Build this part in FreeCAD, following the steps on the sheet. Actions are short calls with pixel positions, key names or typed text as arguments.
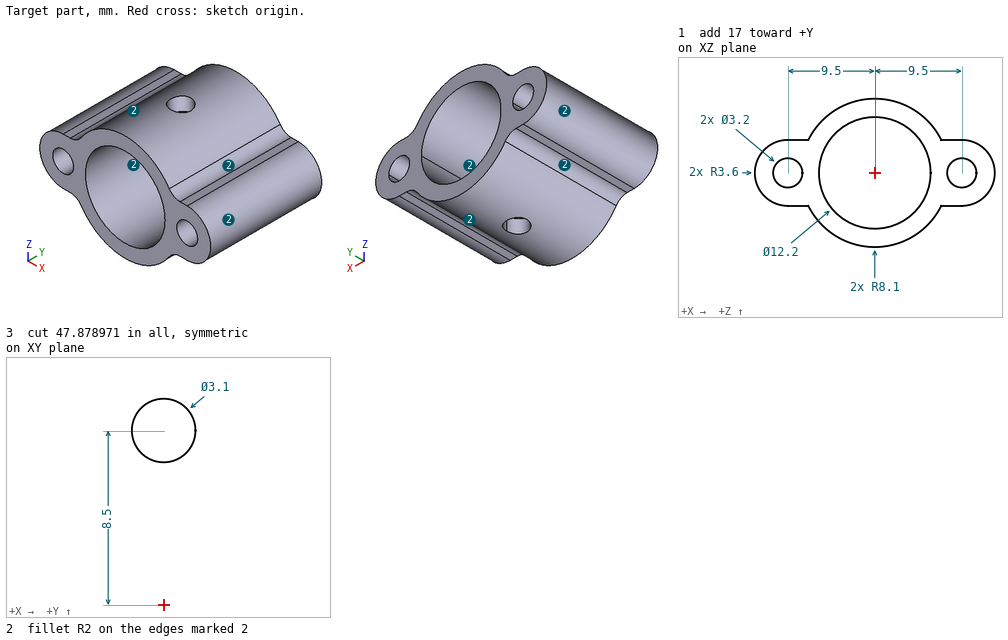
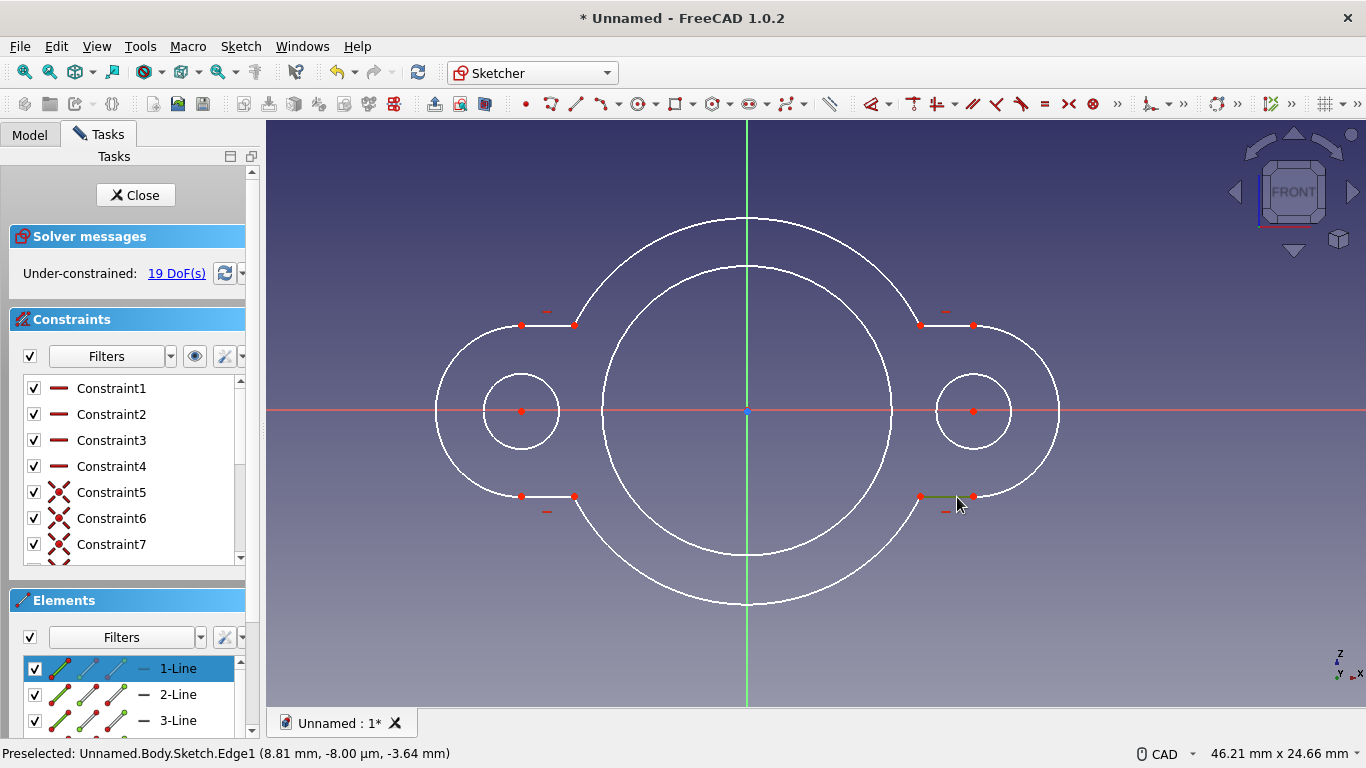
click(1043, 462)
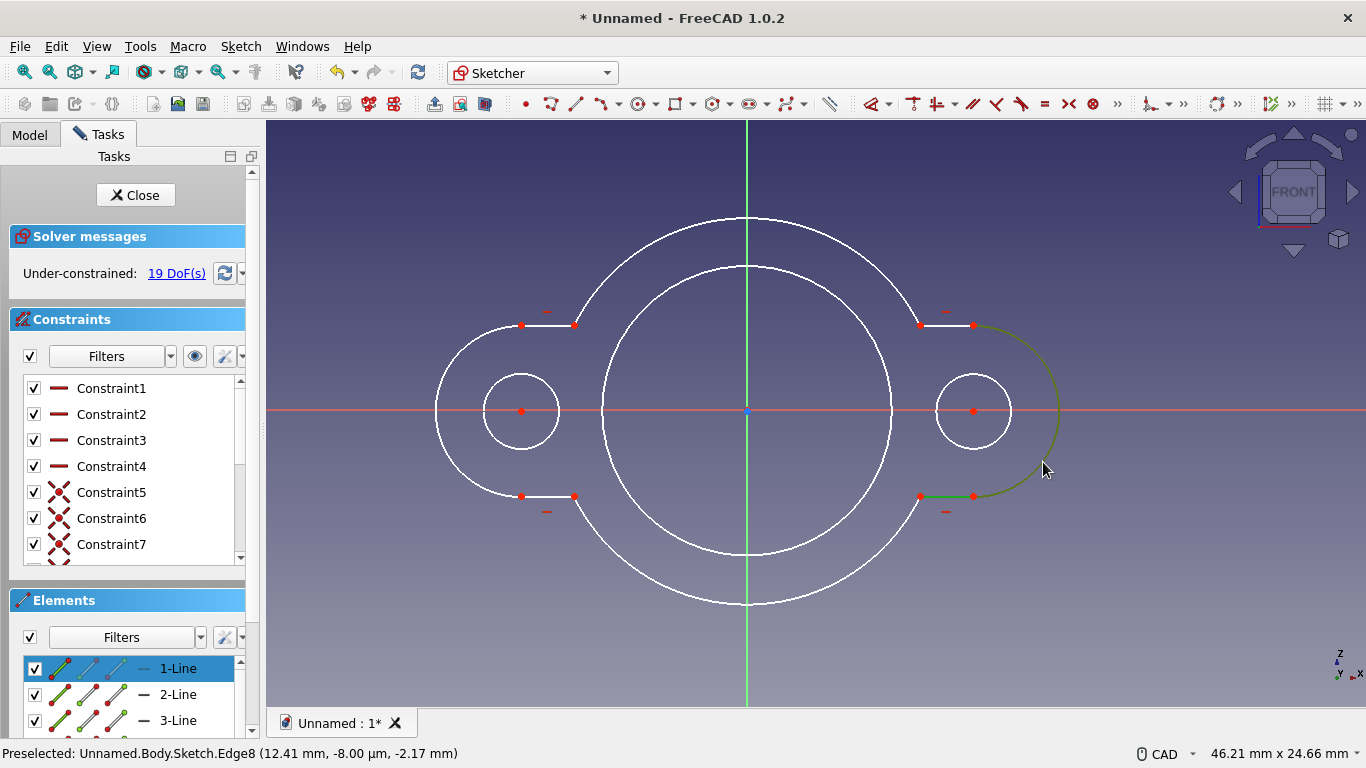
key(t)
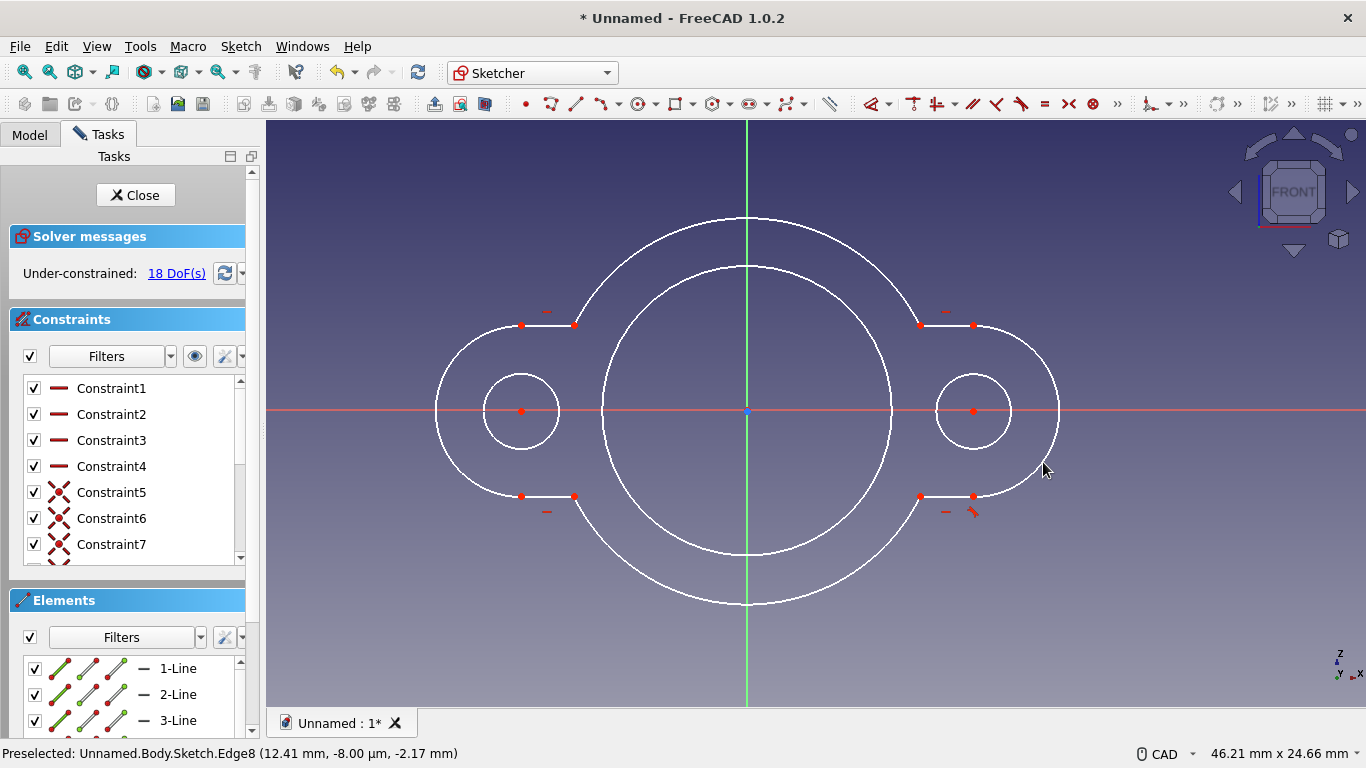
click(558, 497)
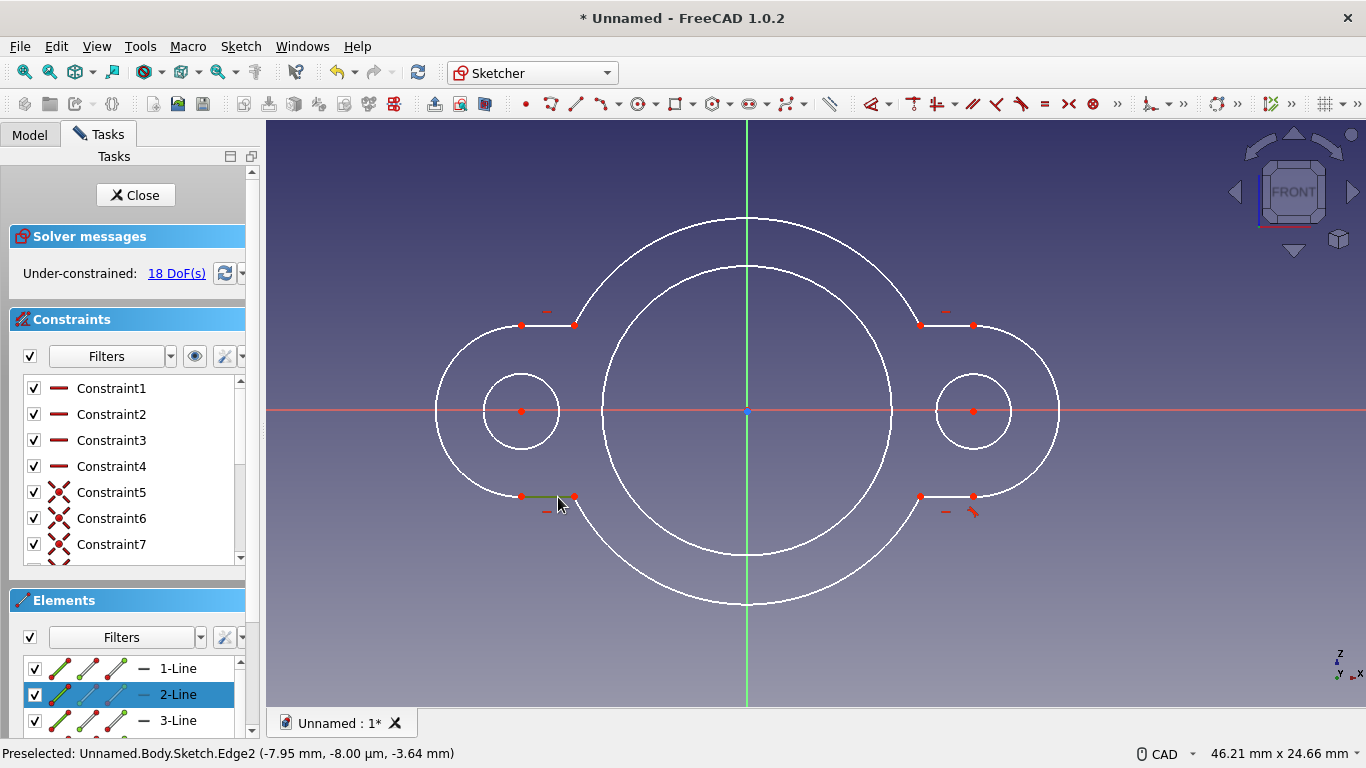
click(452, 361)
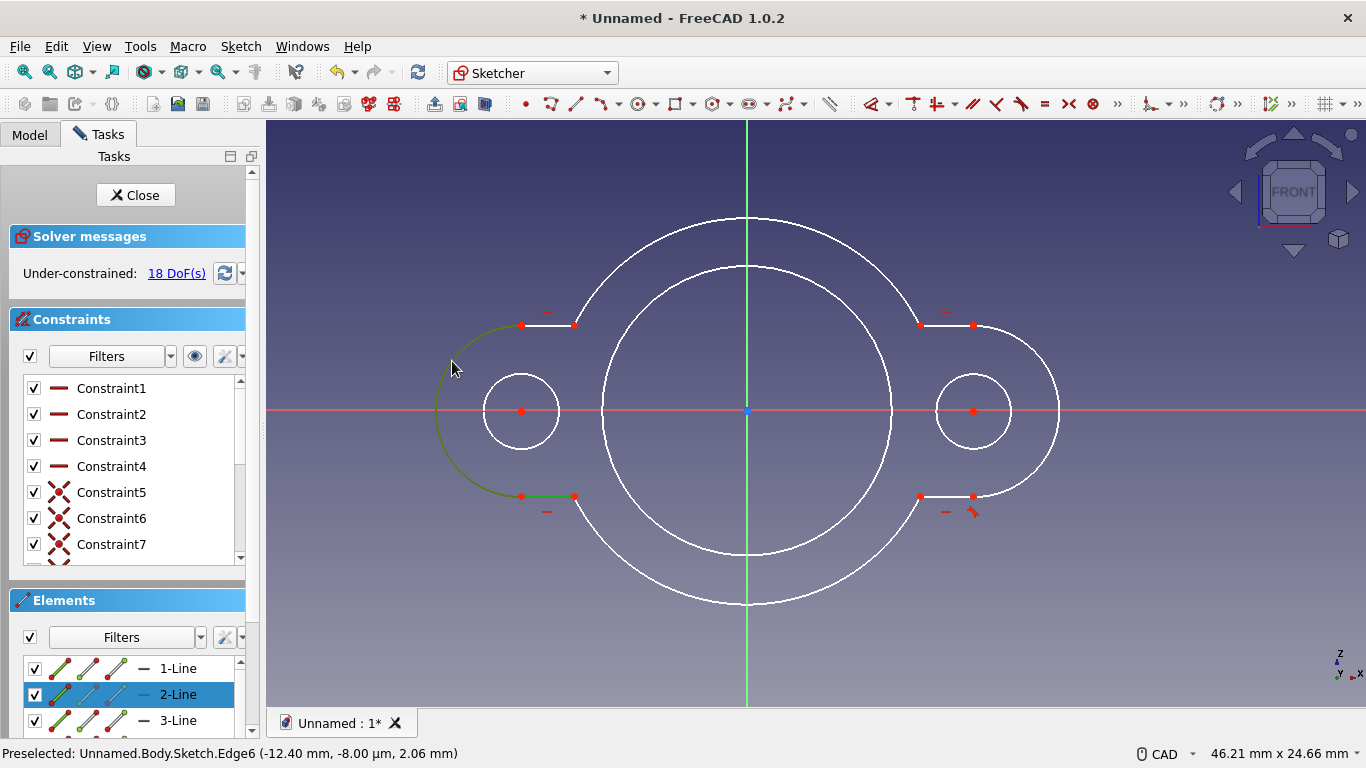
key(t)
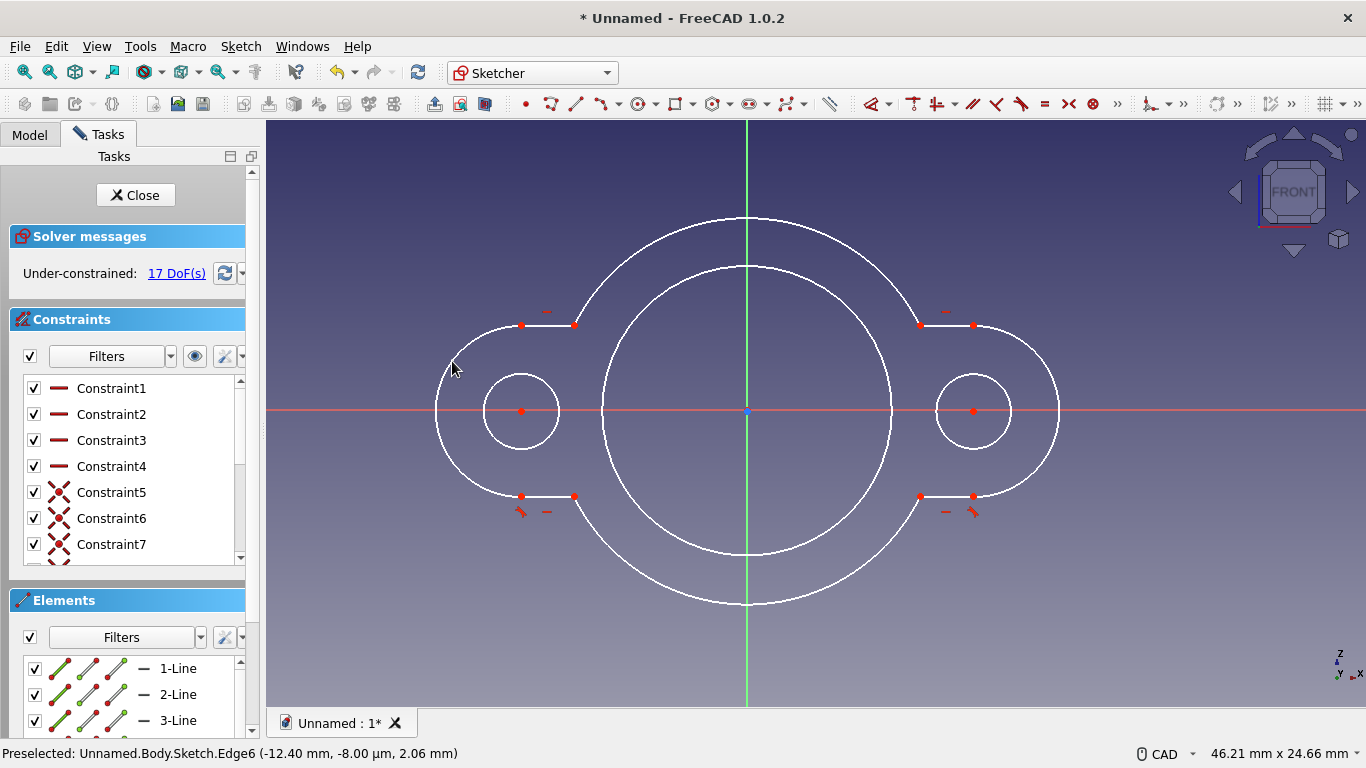
click(537, 326)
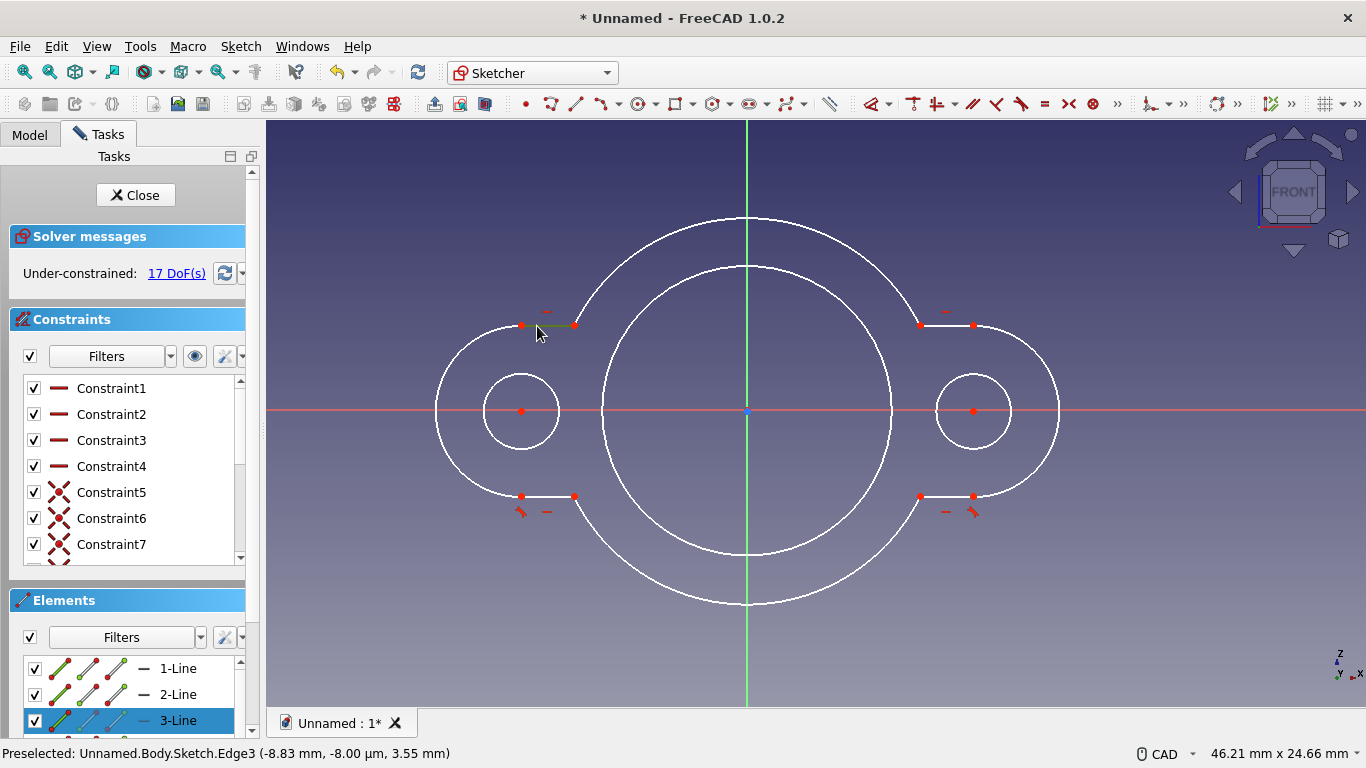
click(452, 361)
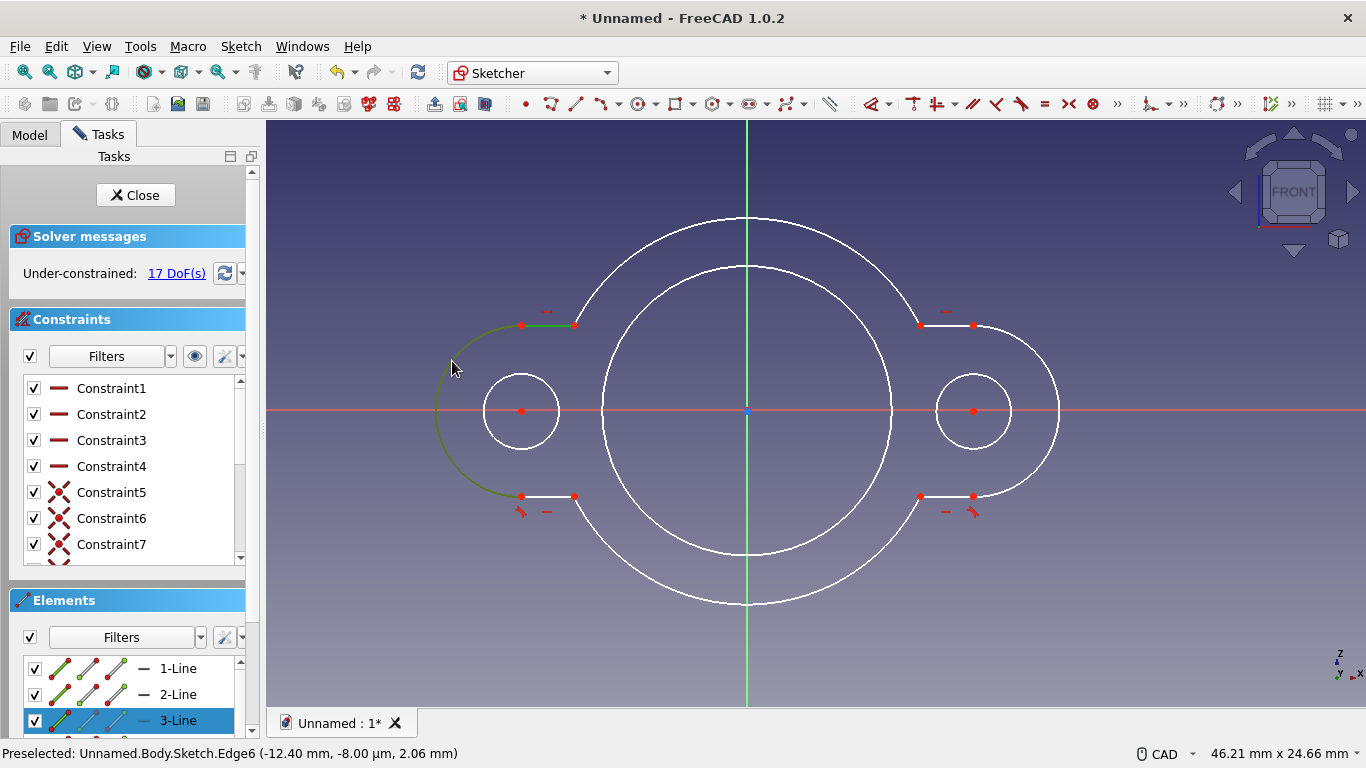
click(1021, 104)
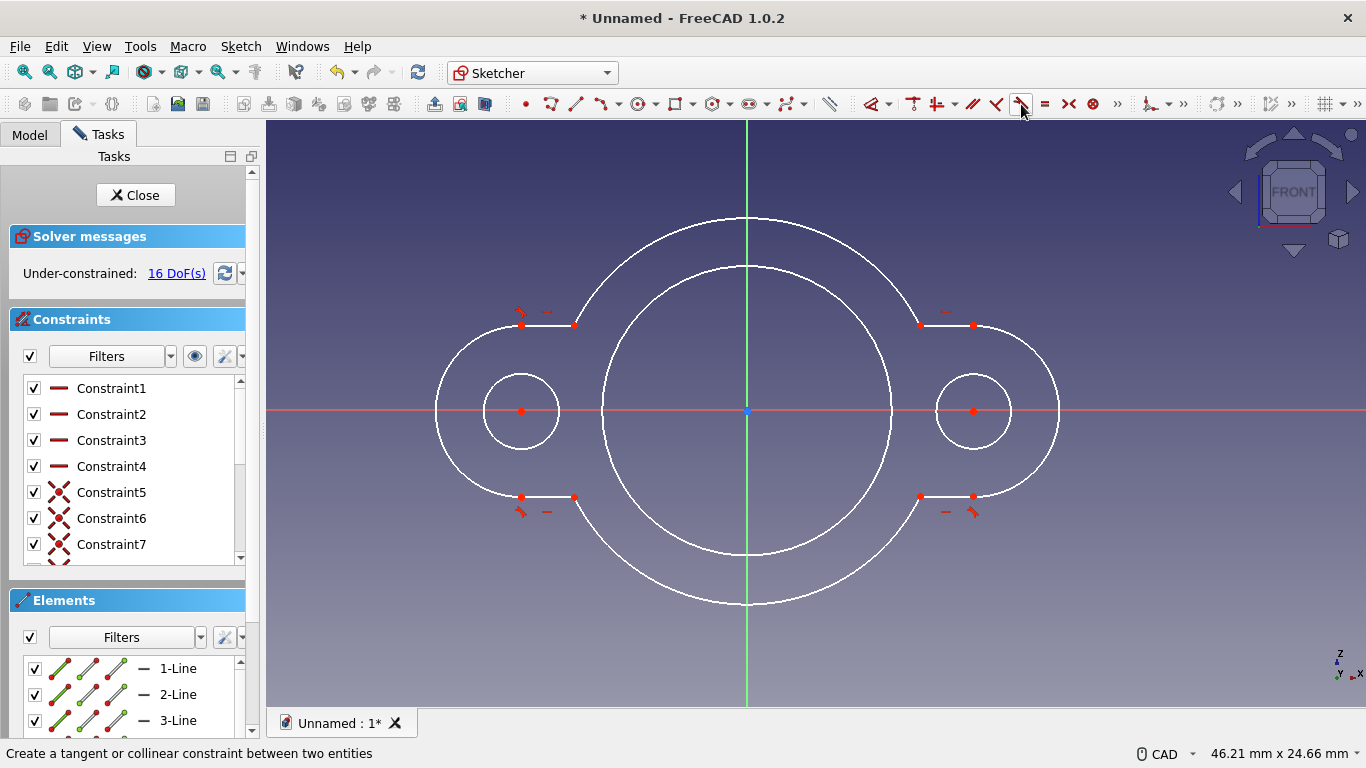
click(936, 326)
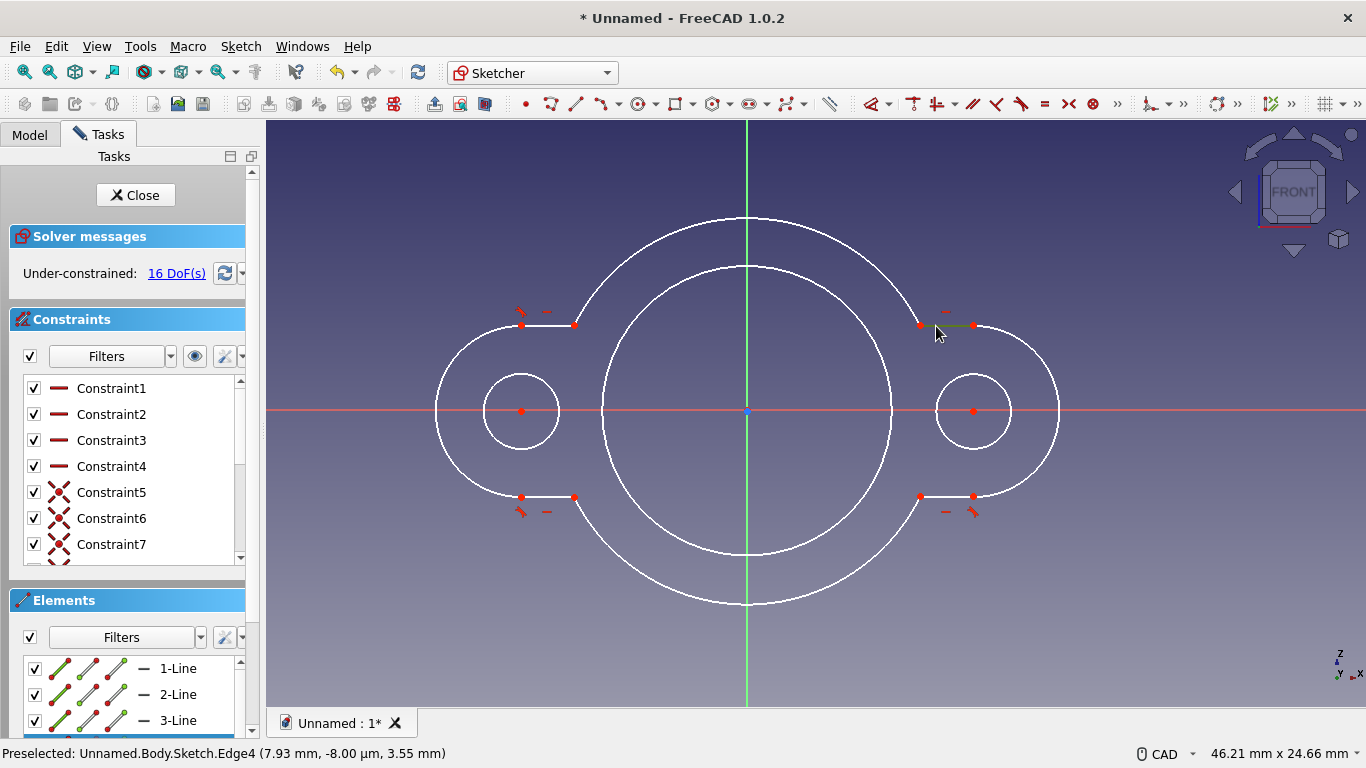
click(1043, 462)